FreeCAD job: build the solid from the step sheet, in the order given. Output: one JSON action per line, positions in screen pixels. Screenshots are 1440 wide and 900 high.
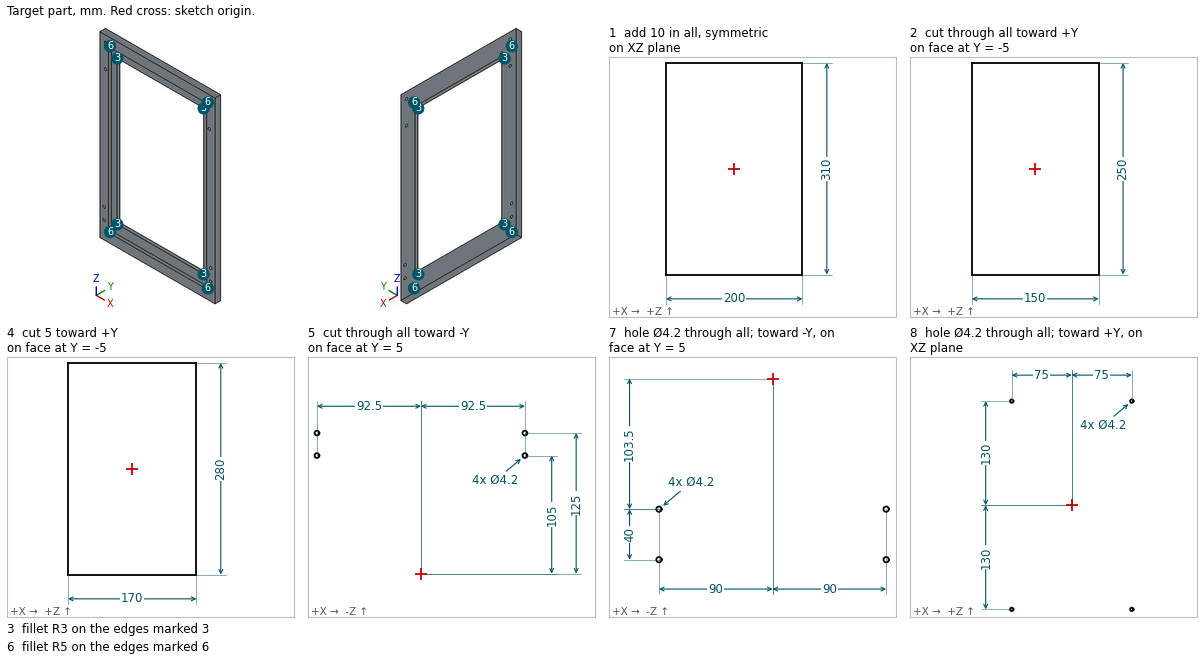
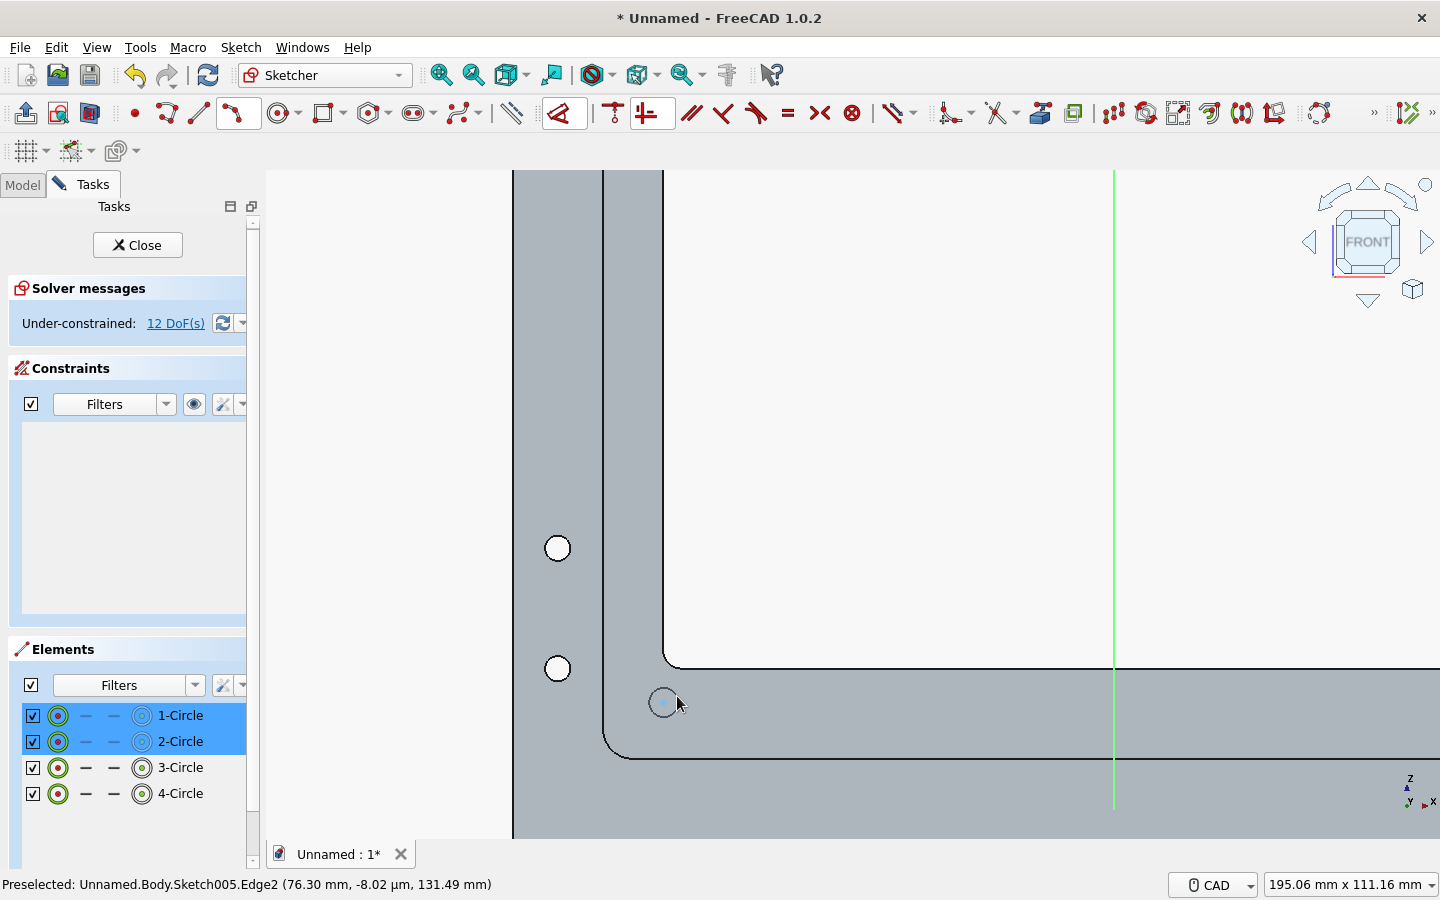
{"action": "left_click", "coordinate": [674, 692]}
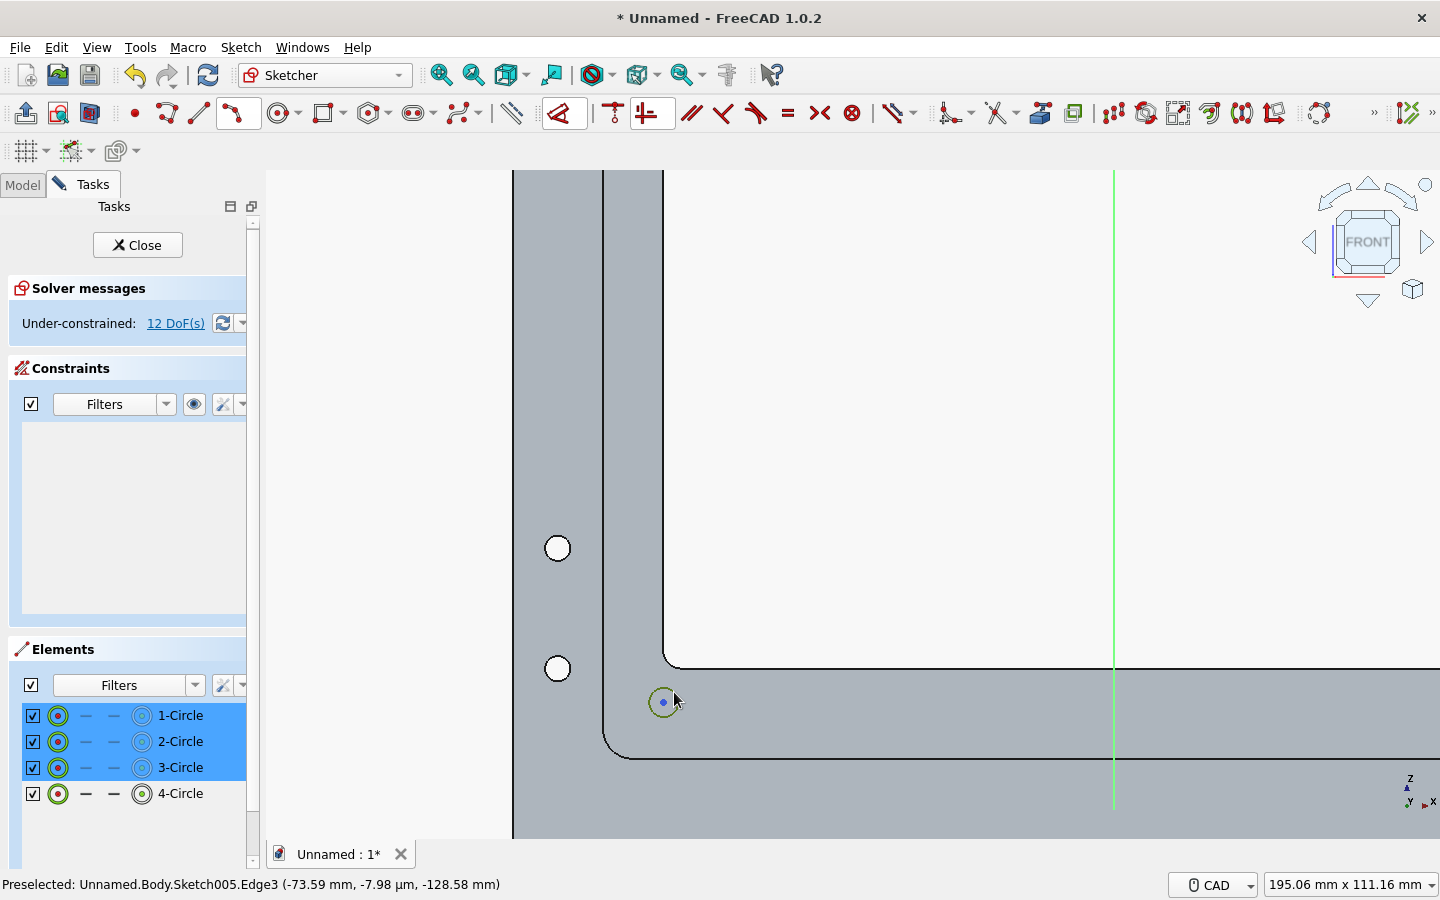
{"action": "scroll", "coordinate": [676, 697], "scroll_direction": "down", "scroll_amount": 7}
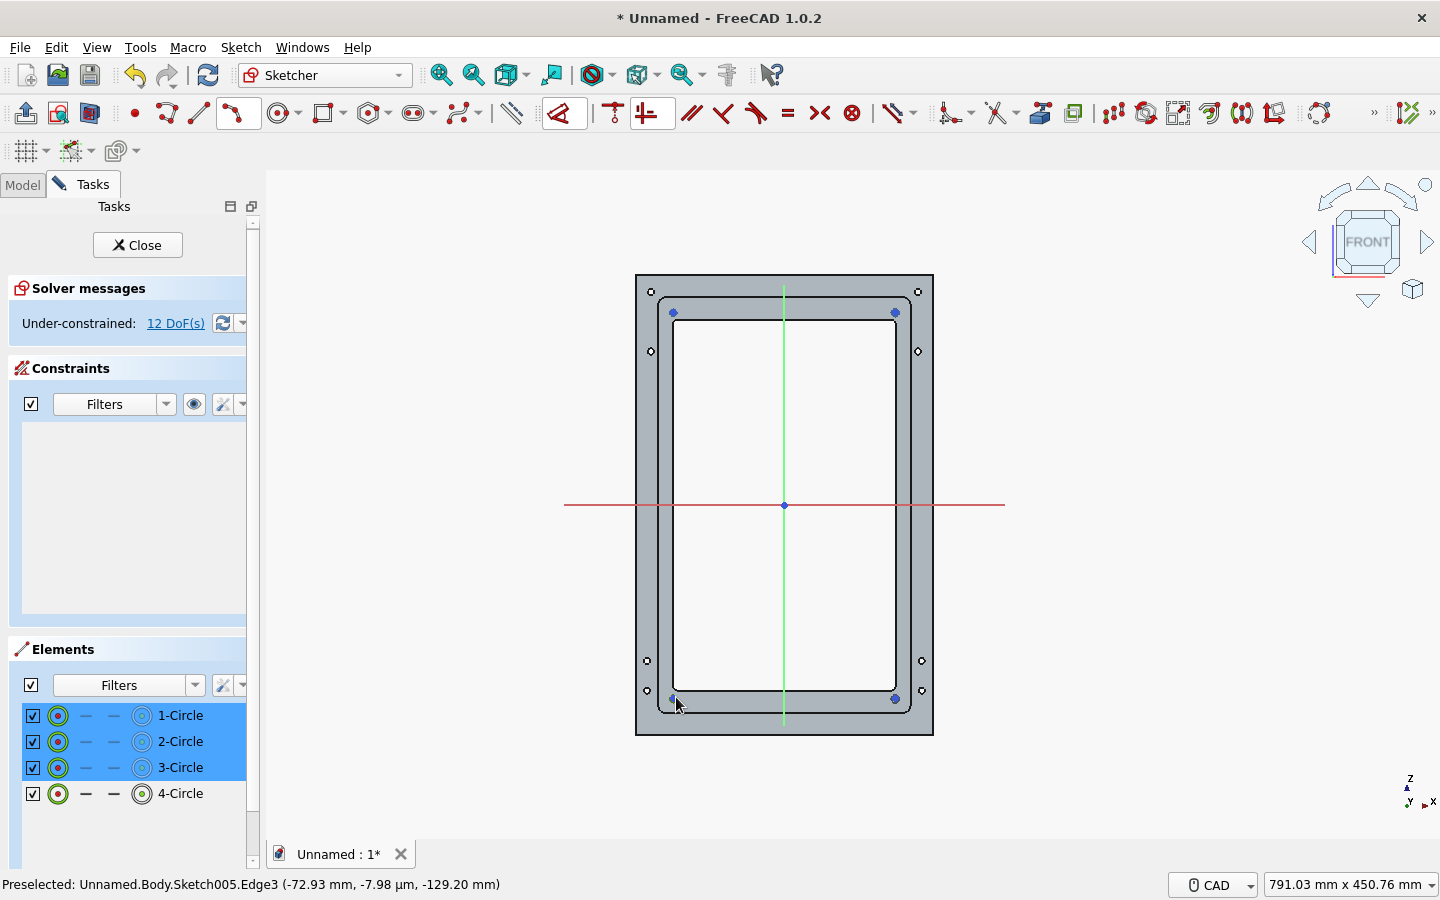
{"action": "scroll", "coordinate": [898, 696], "scroll_direction": "up", "scroll_amount": 7}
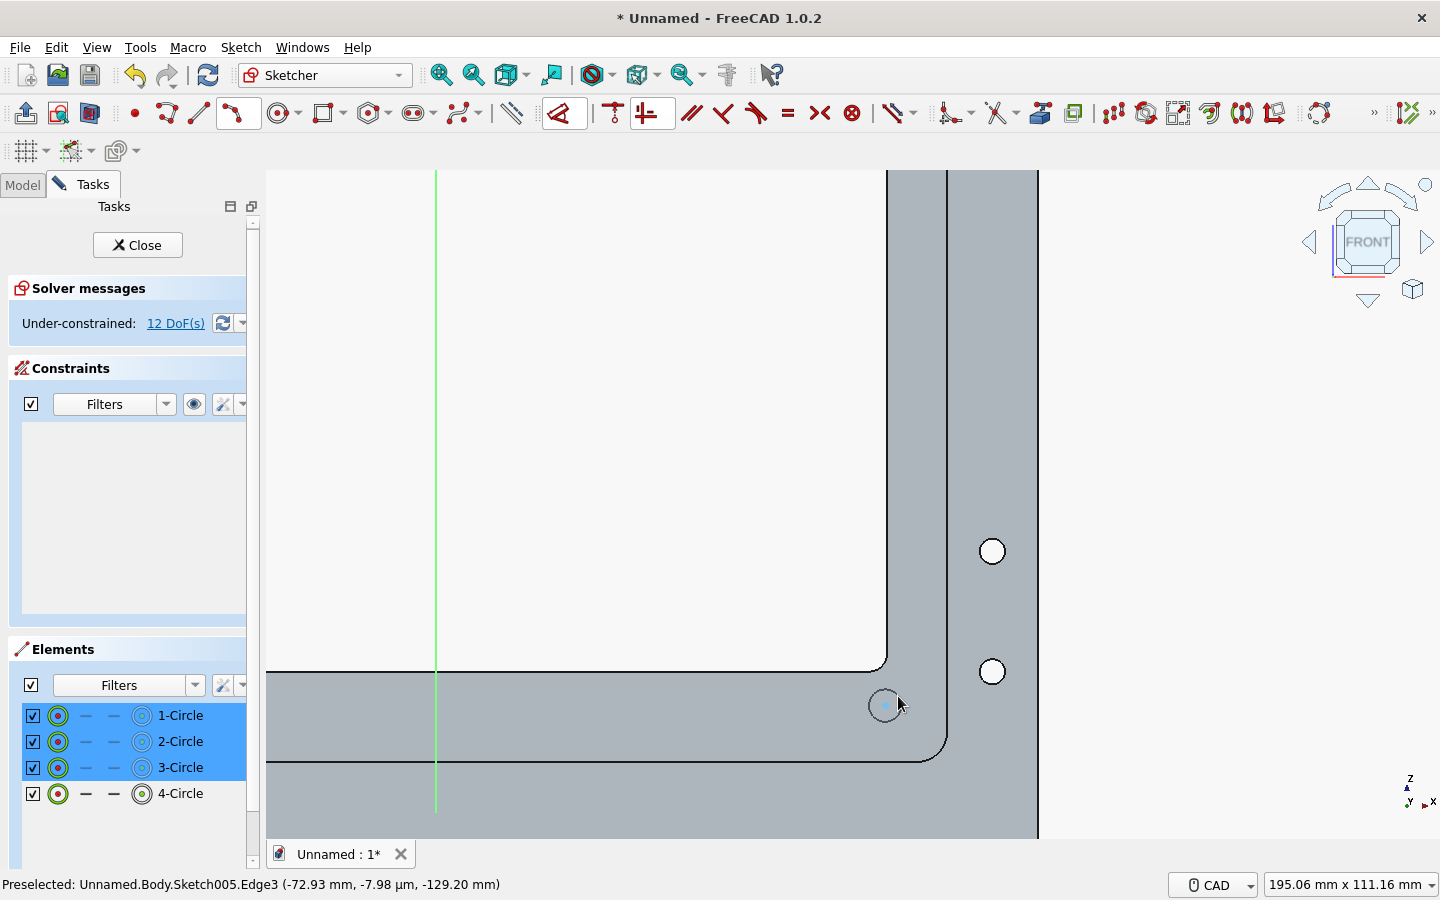
{"action": "left_click", "coordinate": [897, 694]}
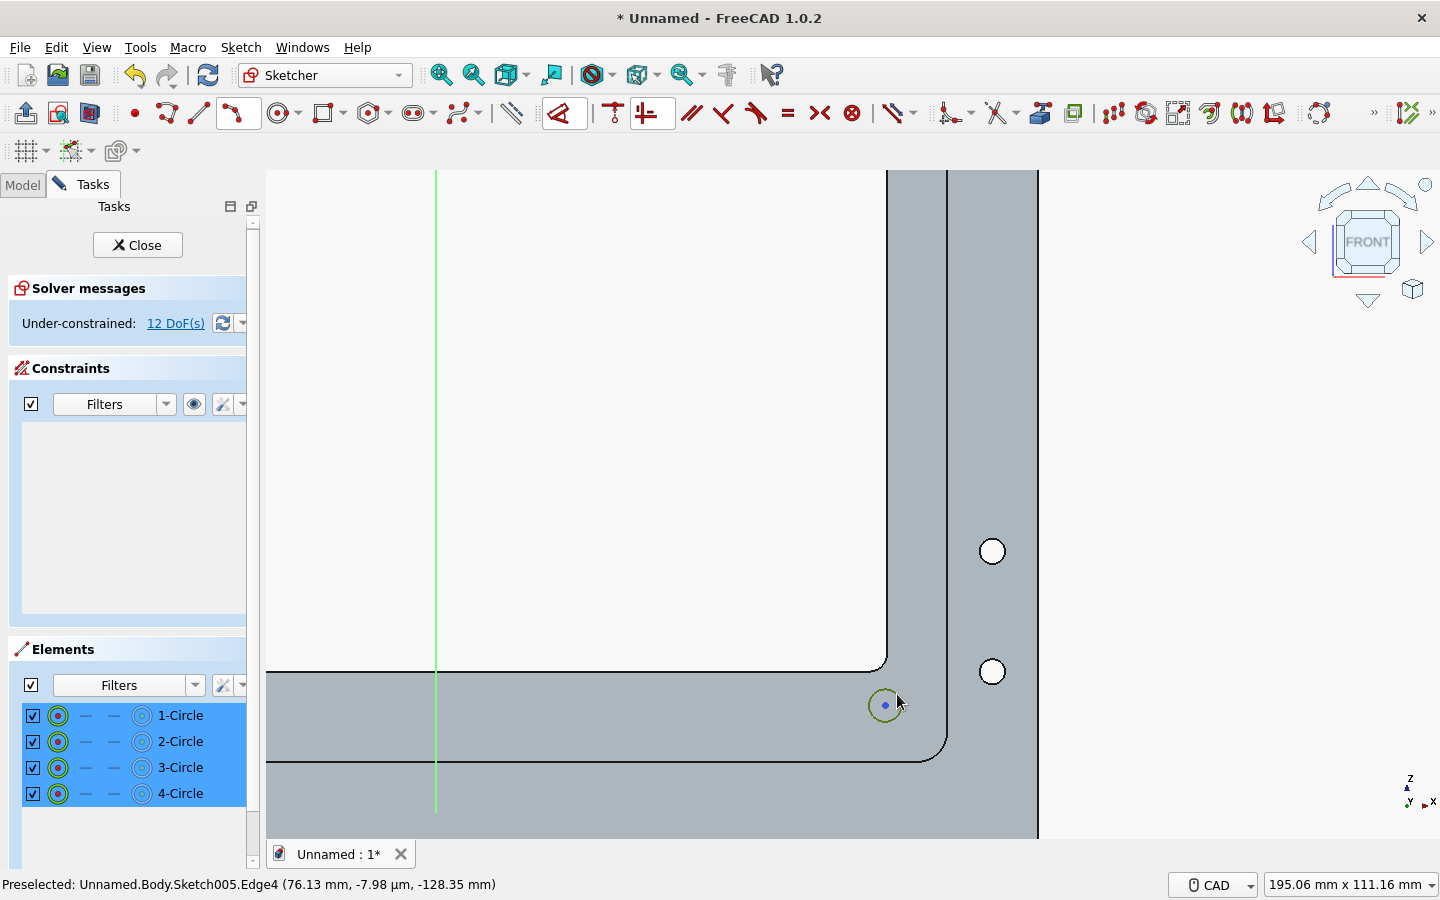
{"action": "left_click", "coordinate": [788, 114]}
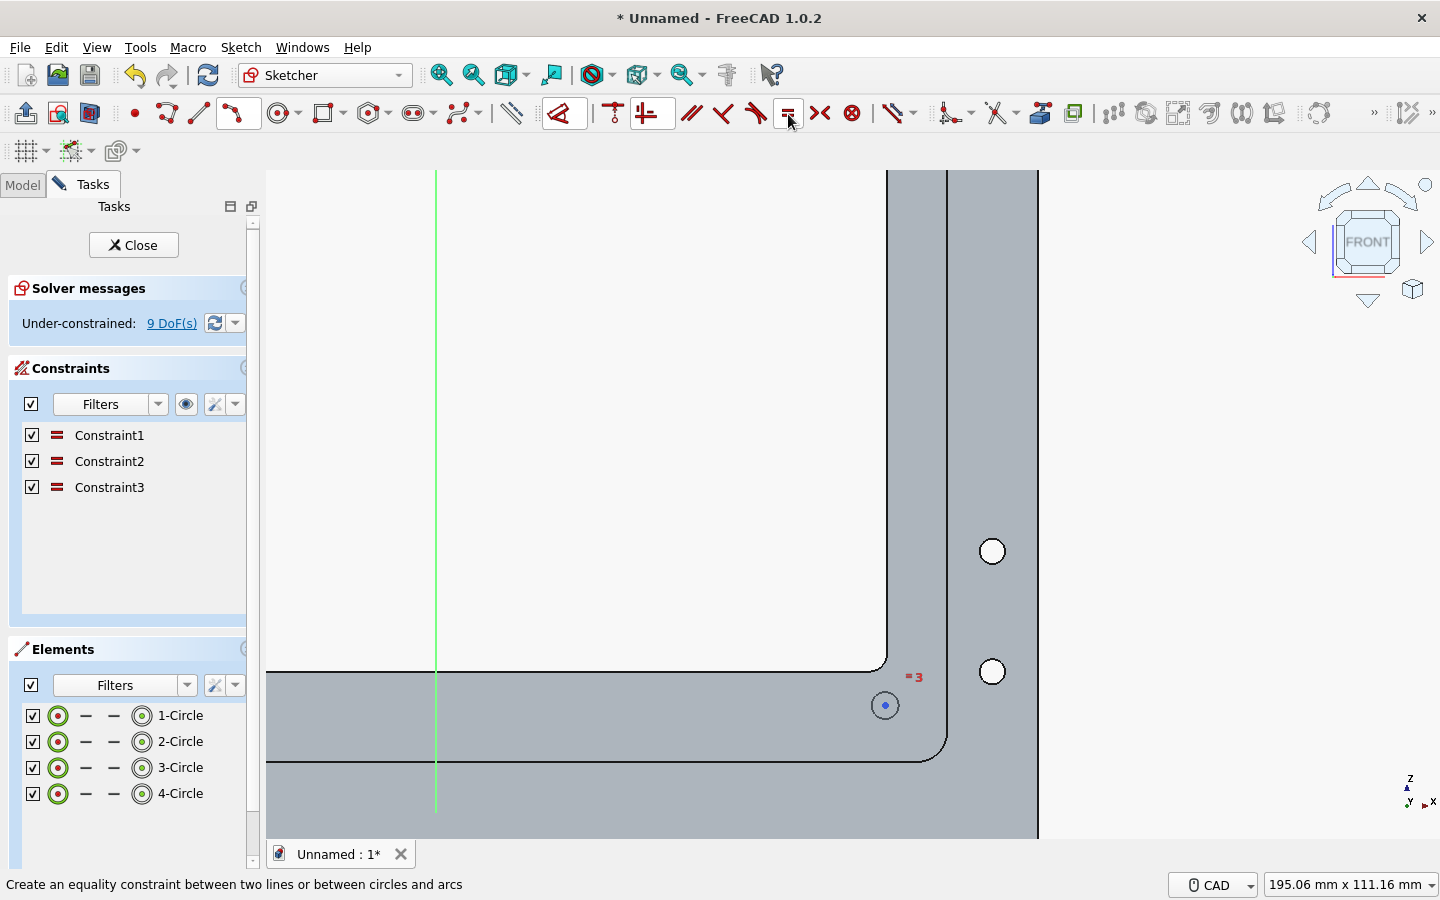
{"action": "scroll", "coordinate": [899, 696], "scroll_direction": "down", "scroll_amount": 7}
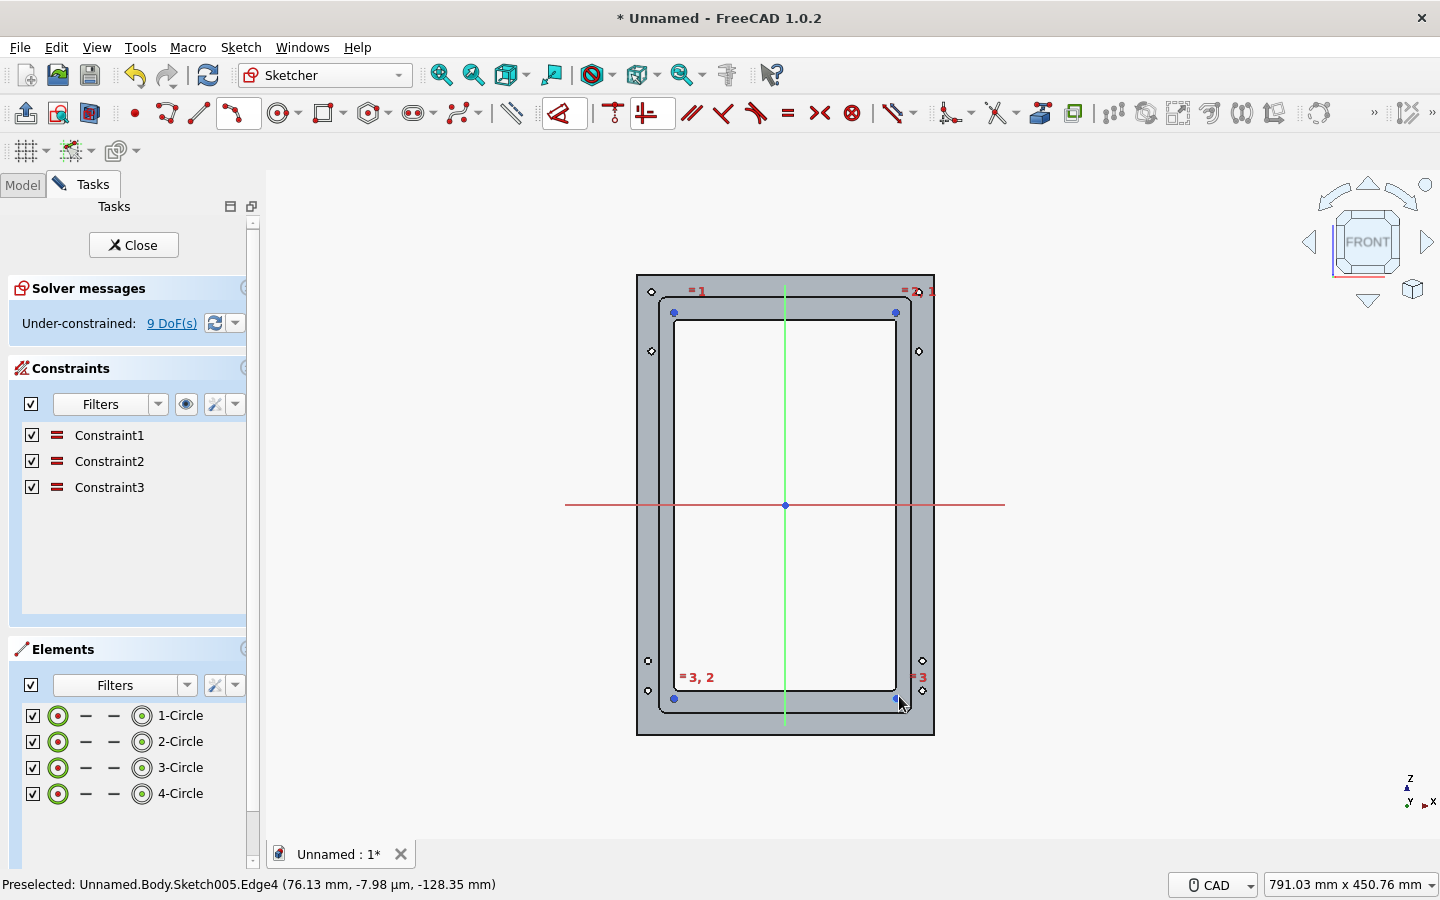
{"action": "left_click", "coordinate": [674, 313]}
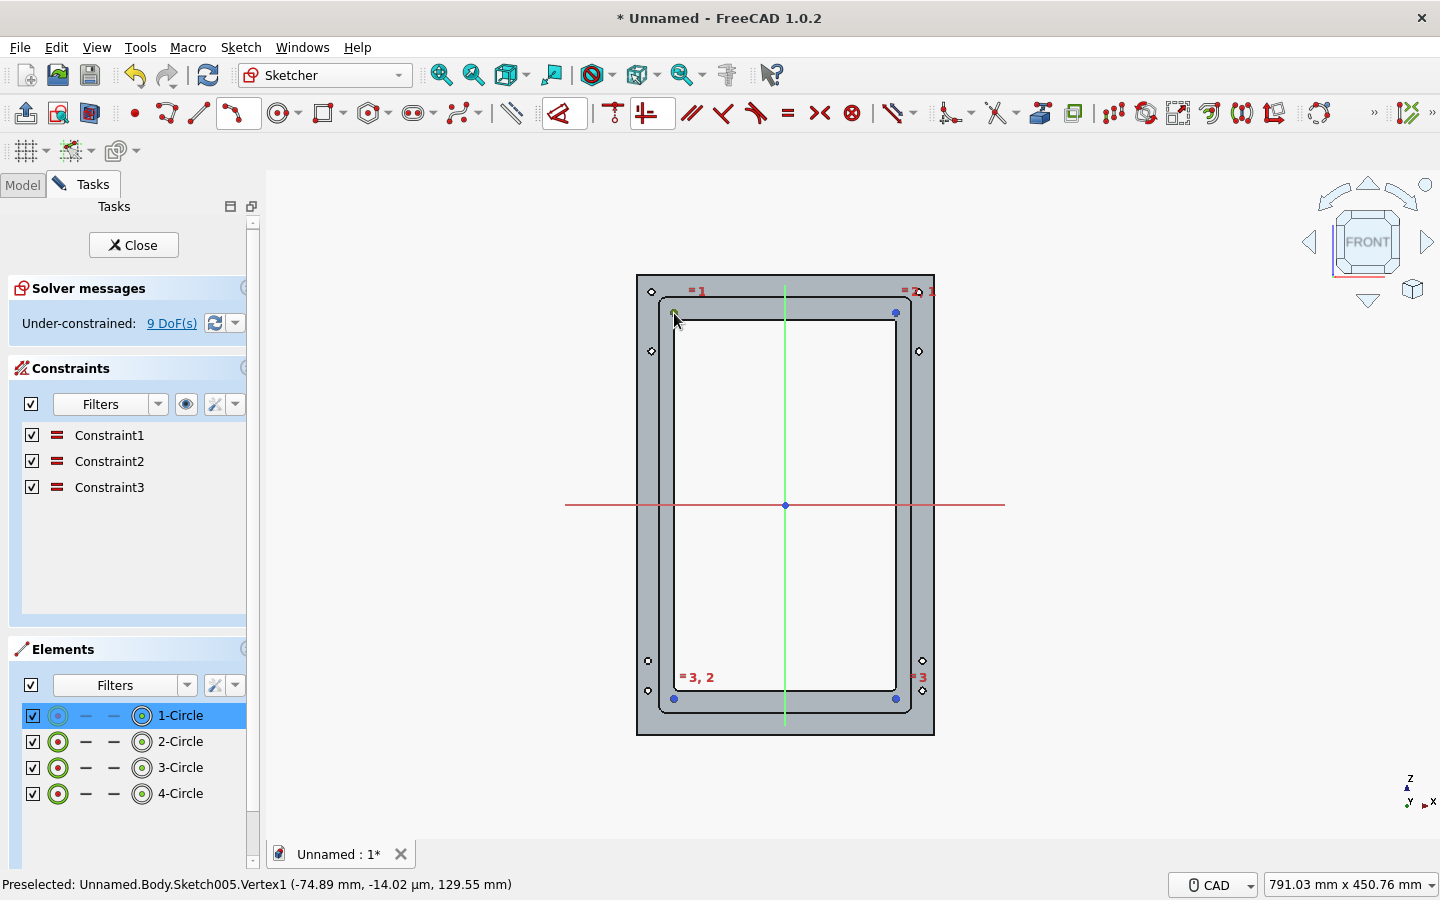
{"action": "left_click", "coordinate": [896, 313]}